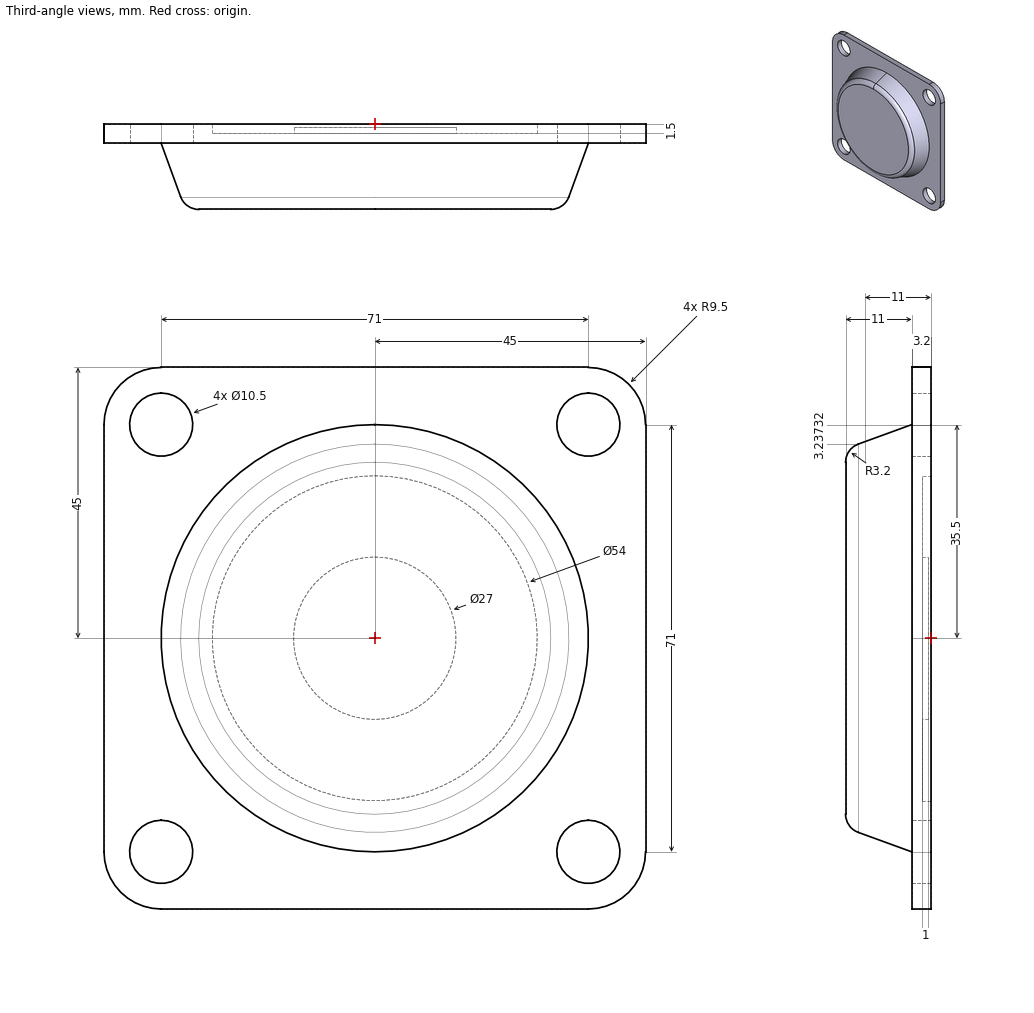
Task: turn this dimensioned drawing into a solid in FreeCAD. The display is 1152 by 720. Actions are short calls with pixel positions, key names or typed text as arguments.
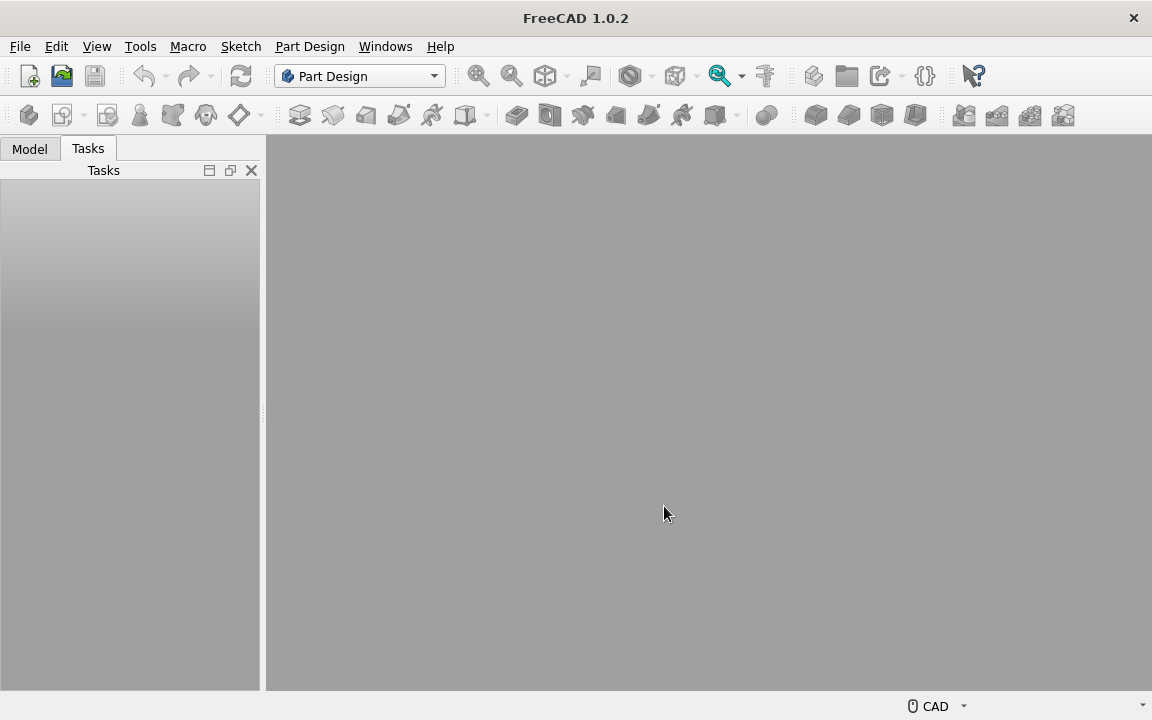
key(ctrl+n)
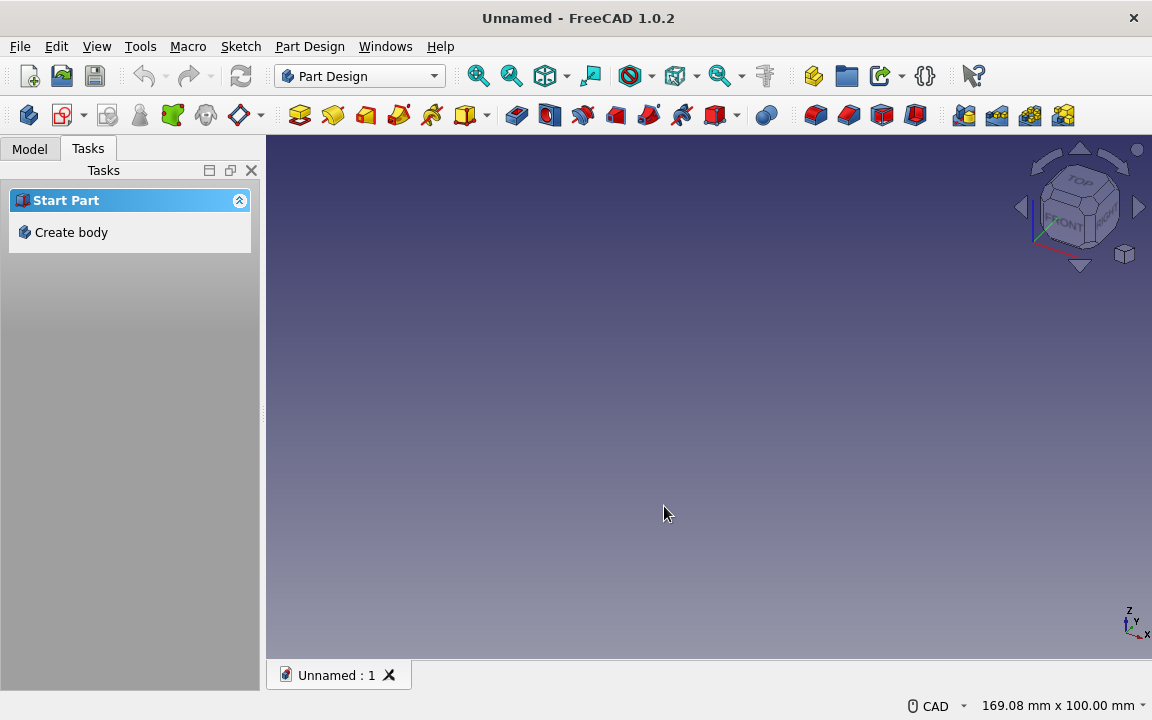
click(62, 116)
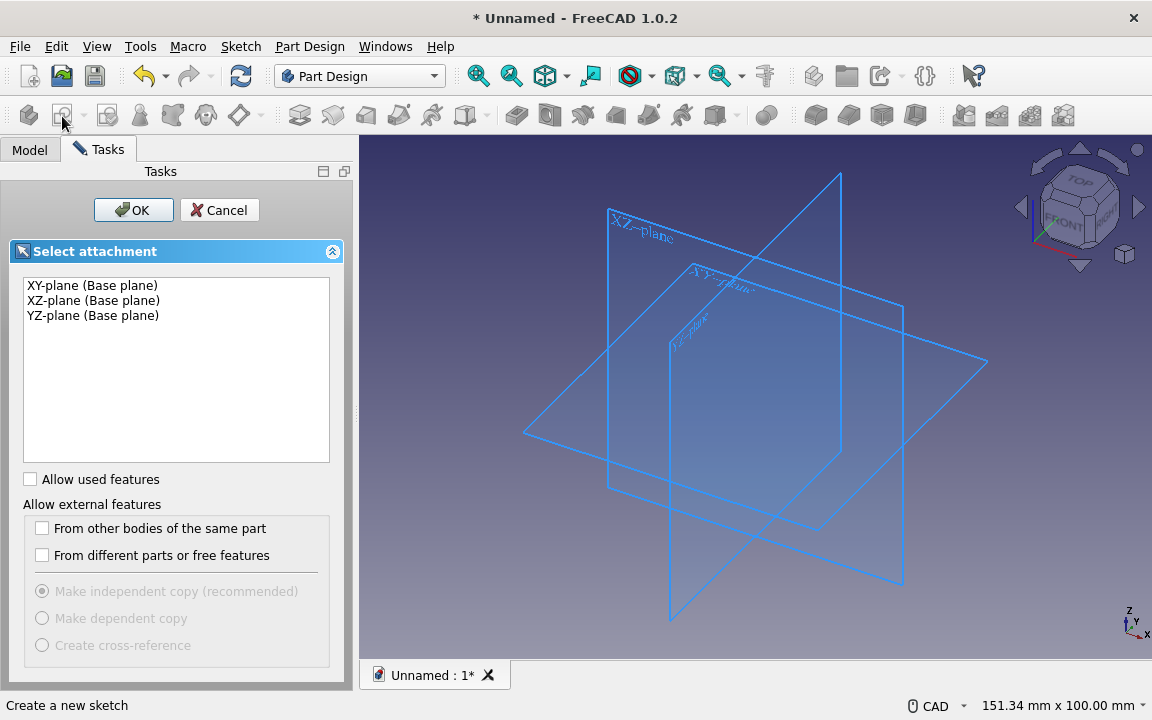
click(84, 300)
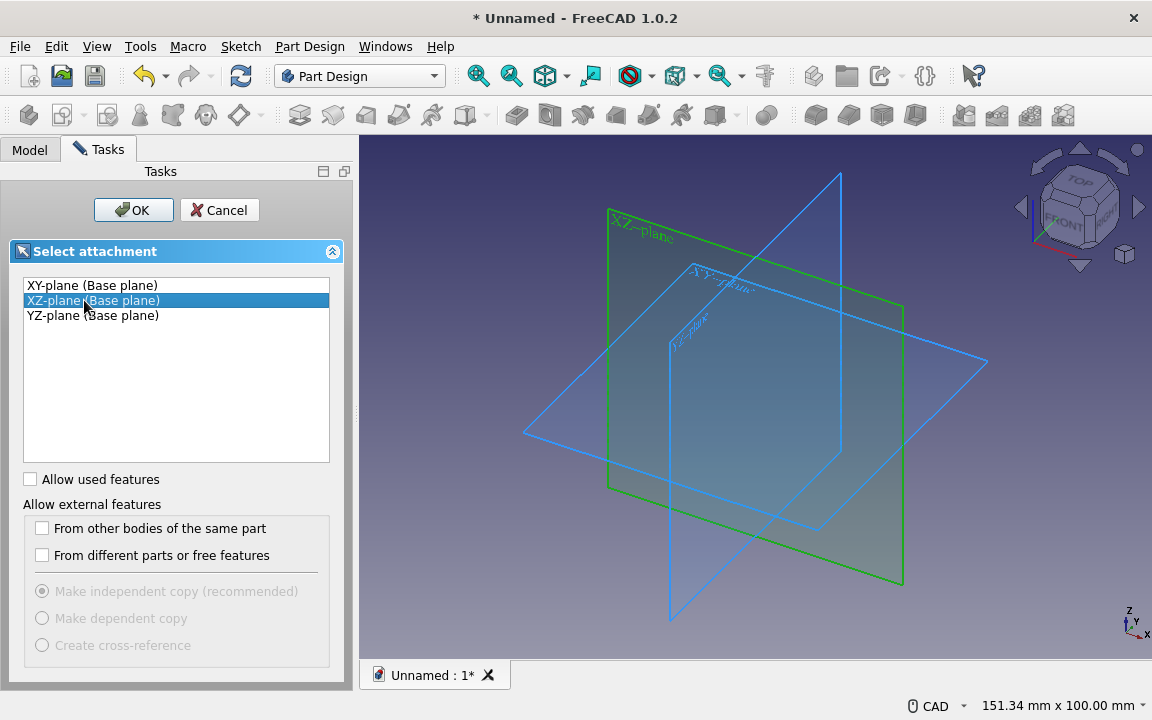
click(134, 210)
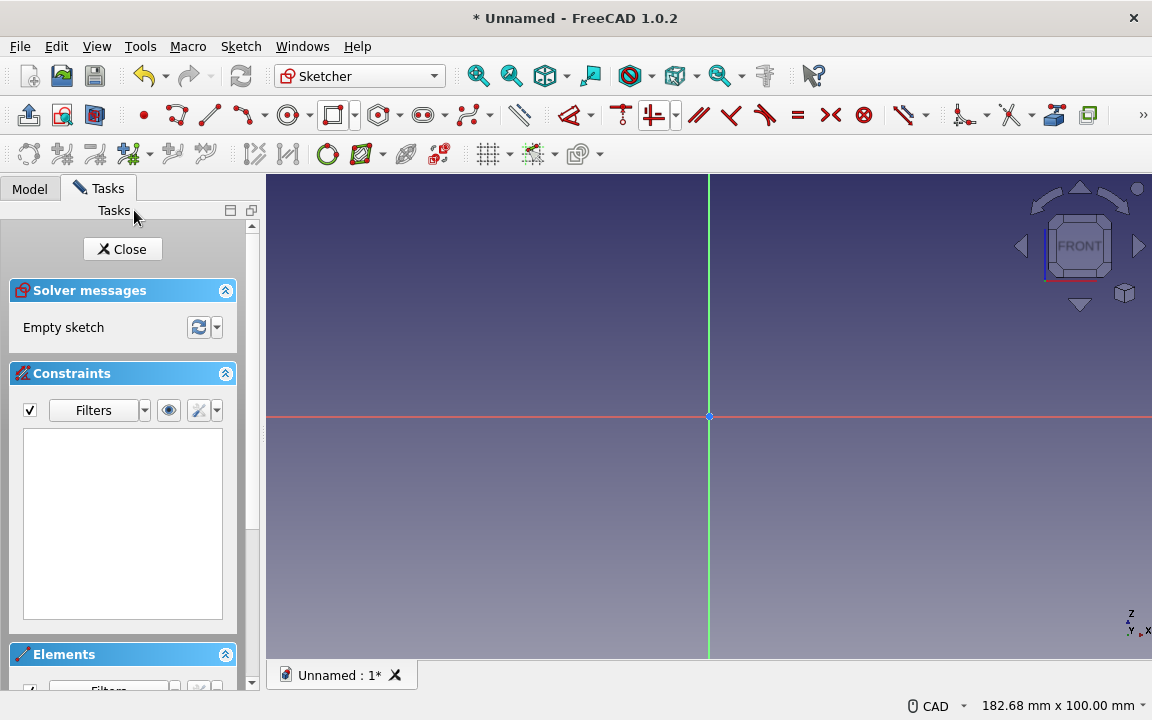
scroll(501, 416, down, 2)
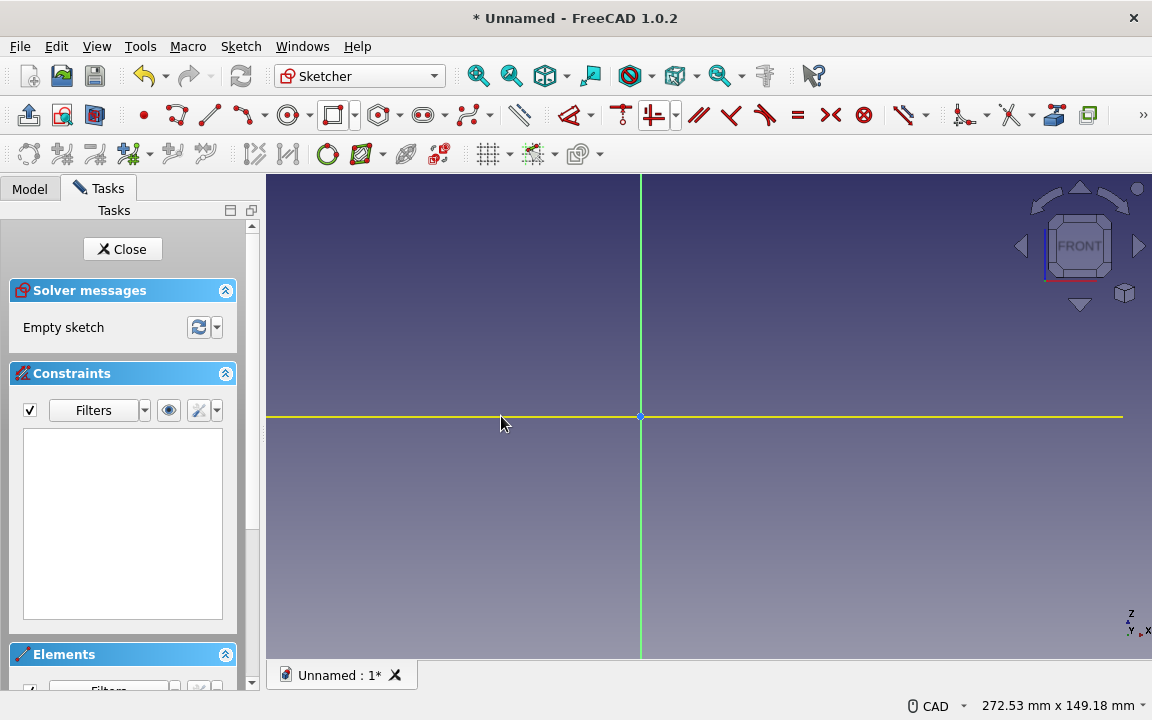
click(210, 116)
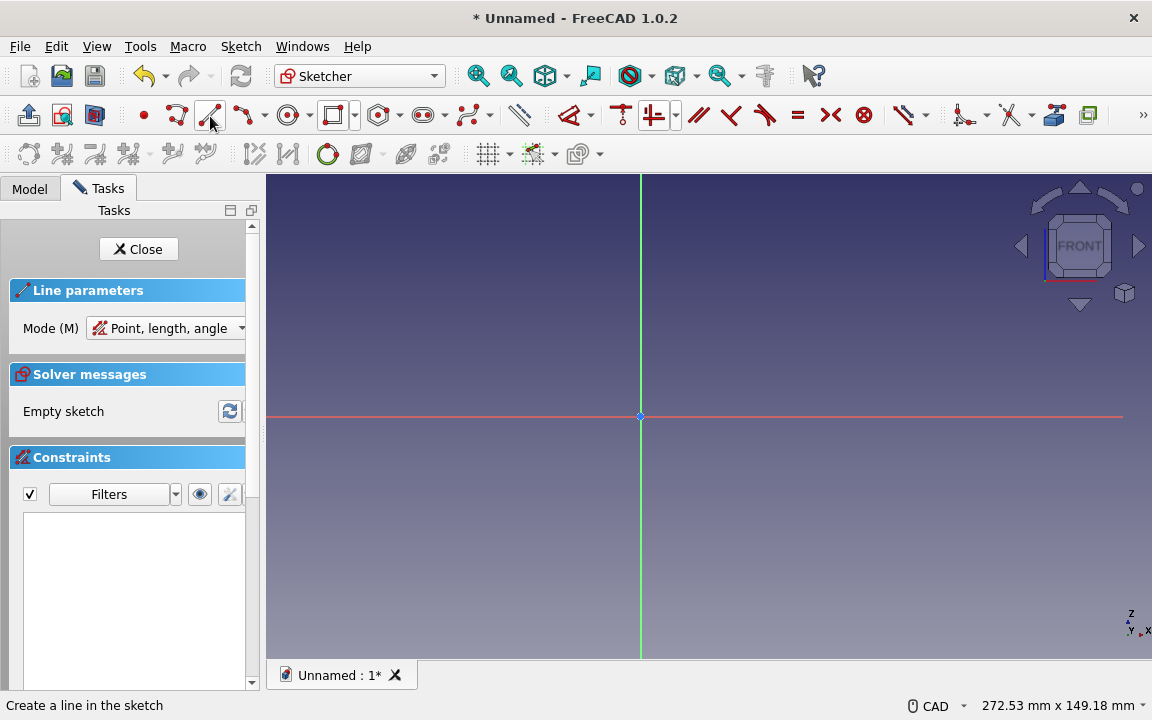
click(525, 270)
click(756, 270)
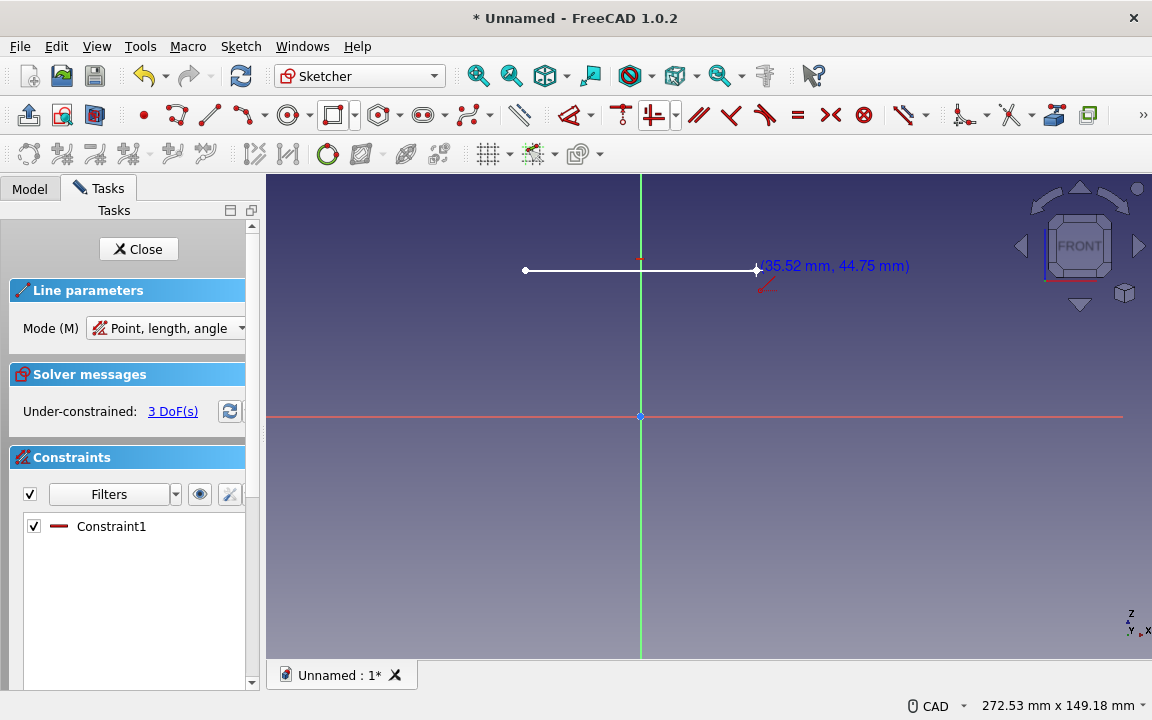
click(787, 301)
click(787, 532)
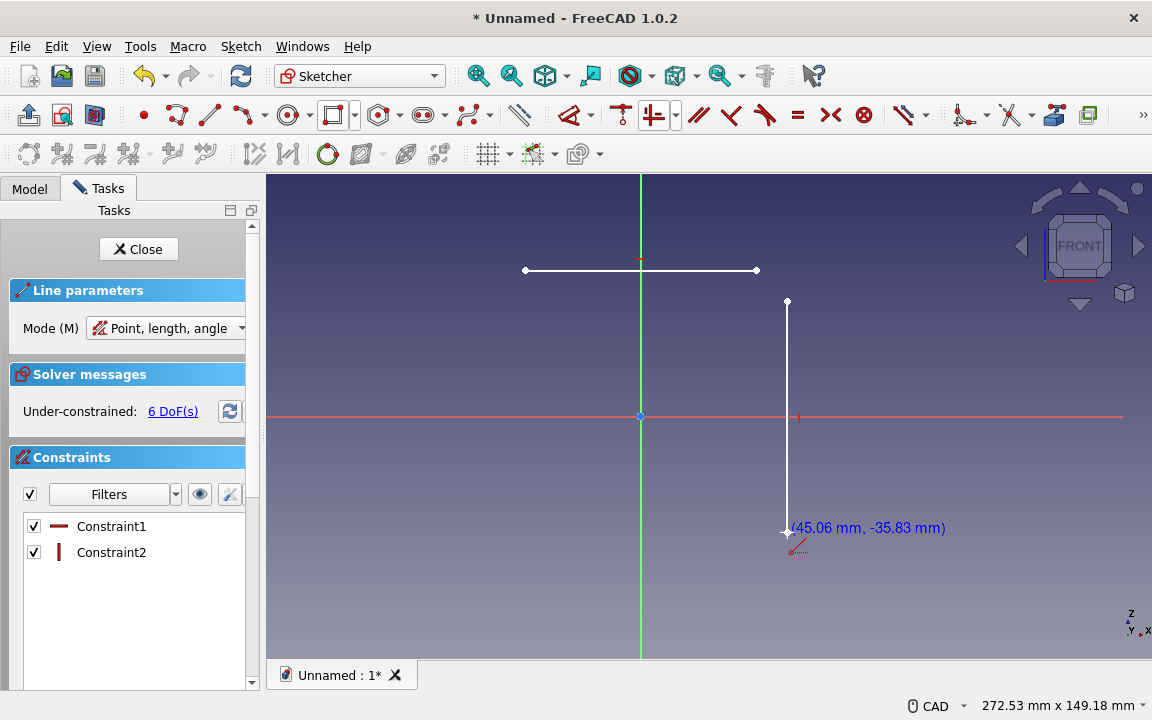
click(756, 563)
click(525, 563)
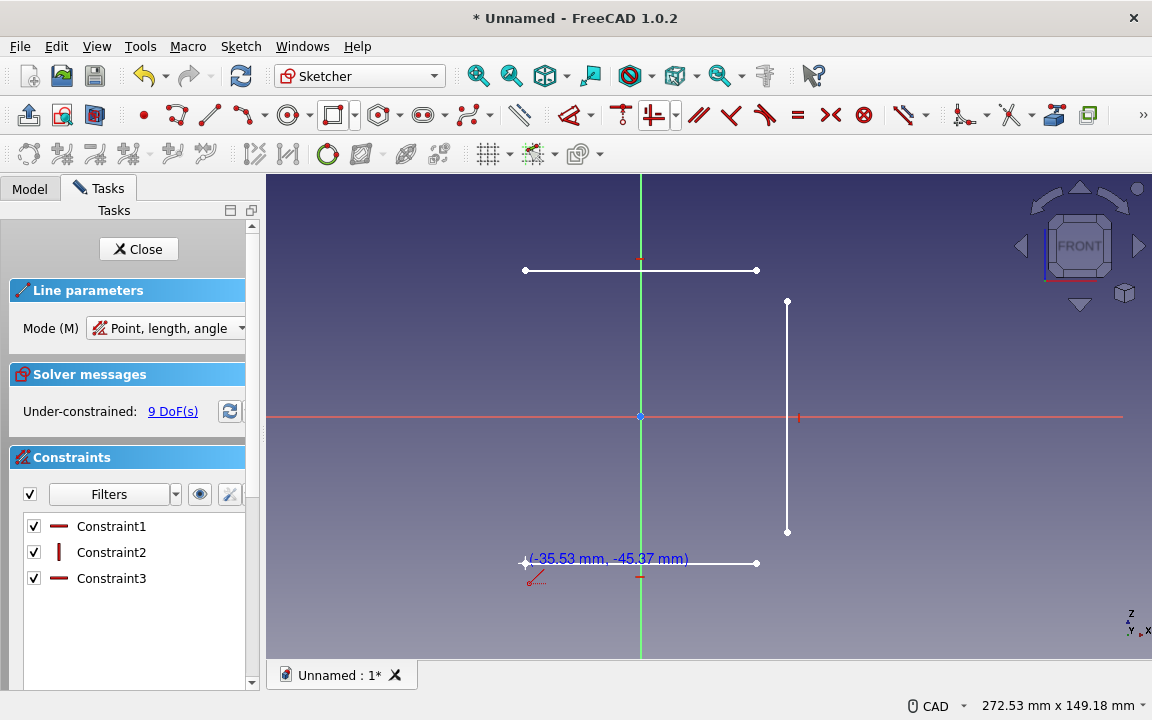
click(494, 532)
click(494, 301)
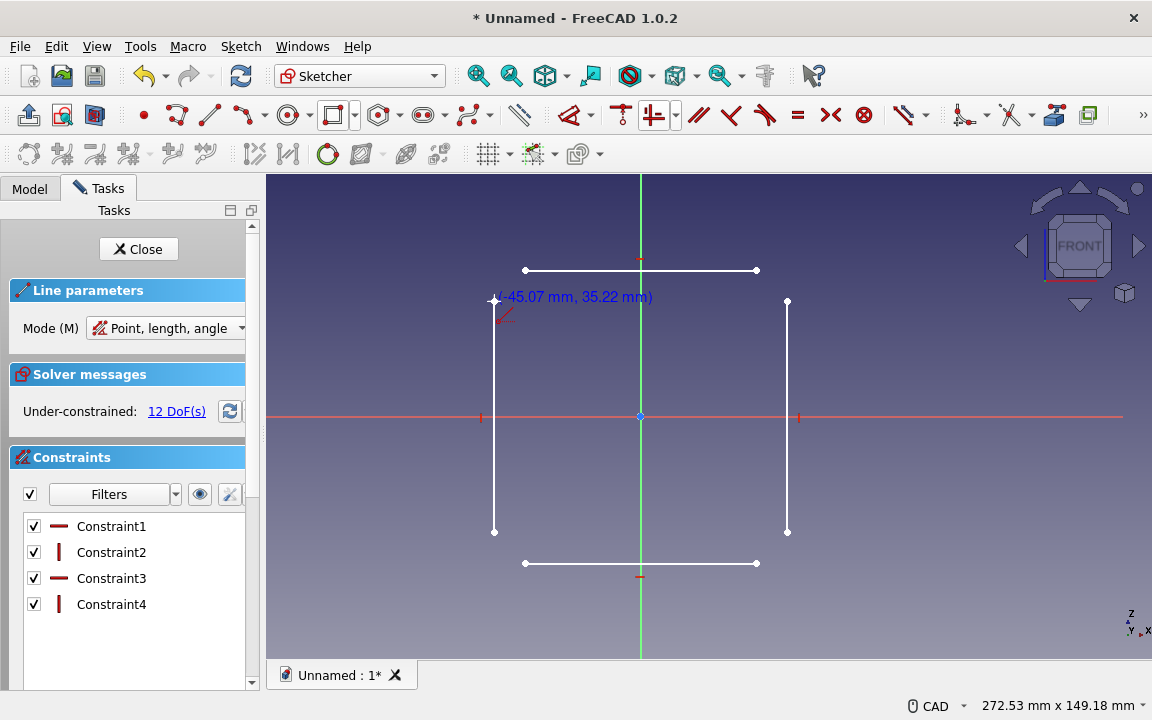
key(g)
key(3)
key(a)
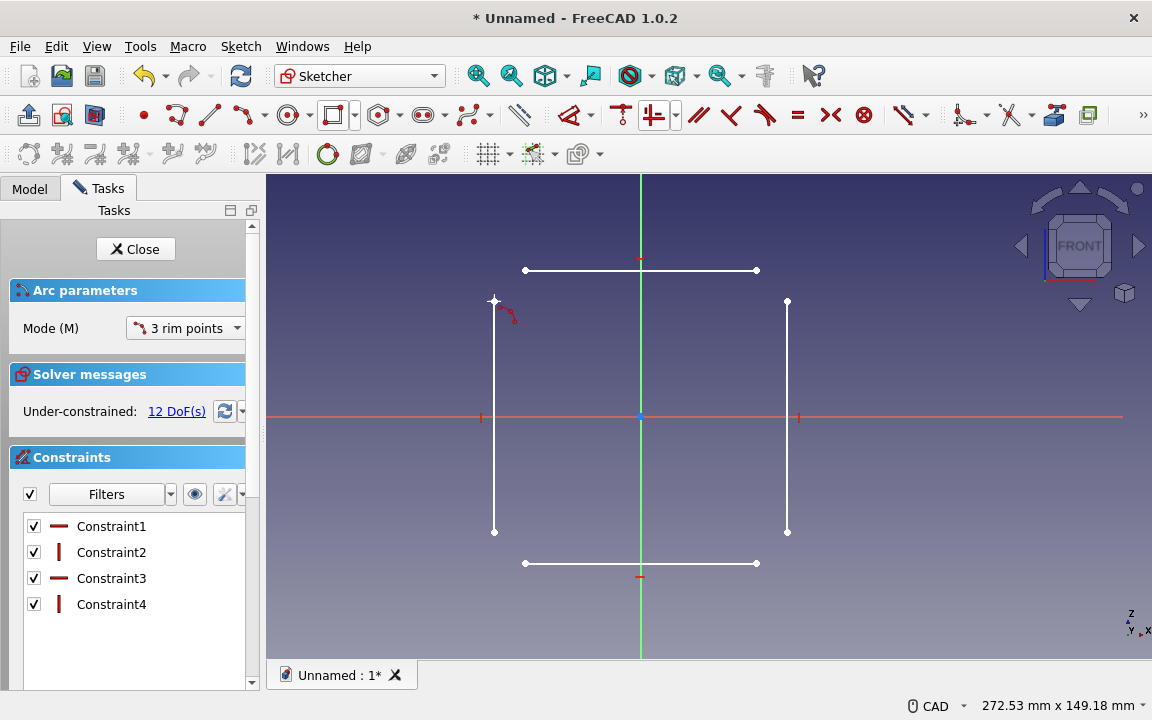
click(756, 271)
click(787, 302)